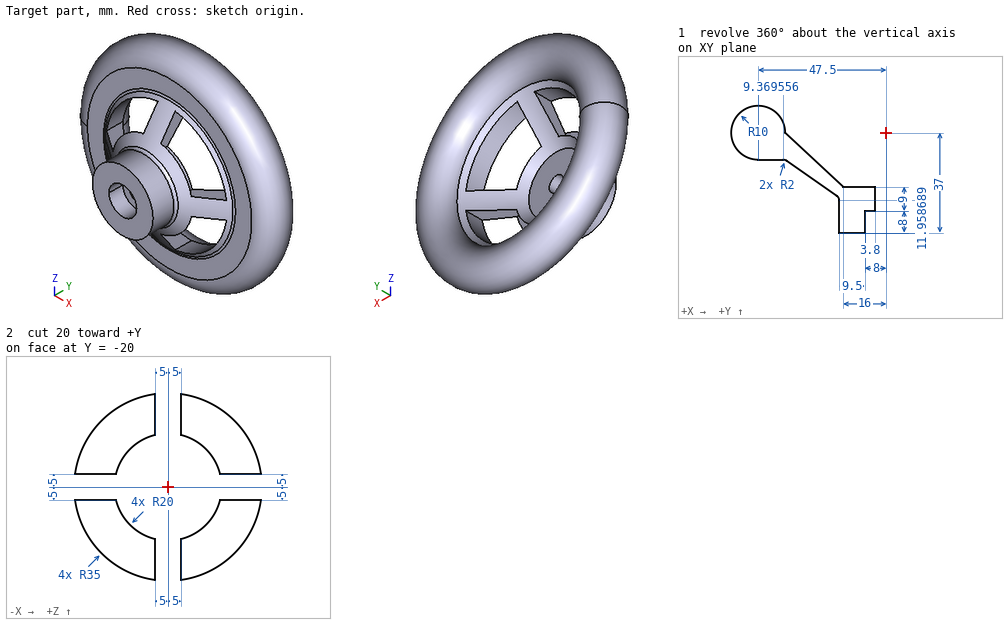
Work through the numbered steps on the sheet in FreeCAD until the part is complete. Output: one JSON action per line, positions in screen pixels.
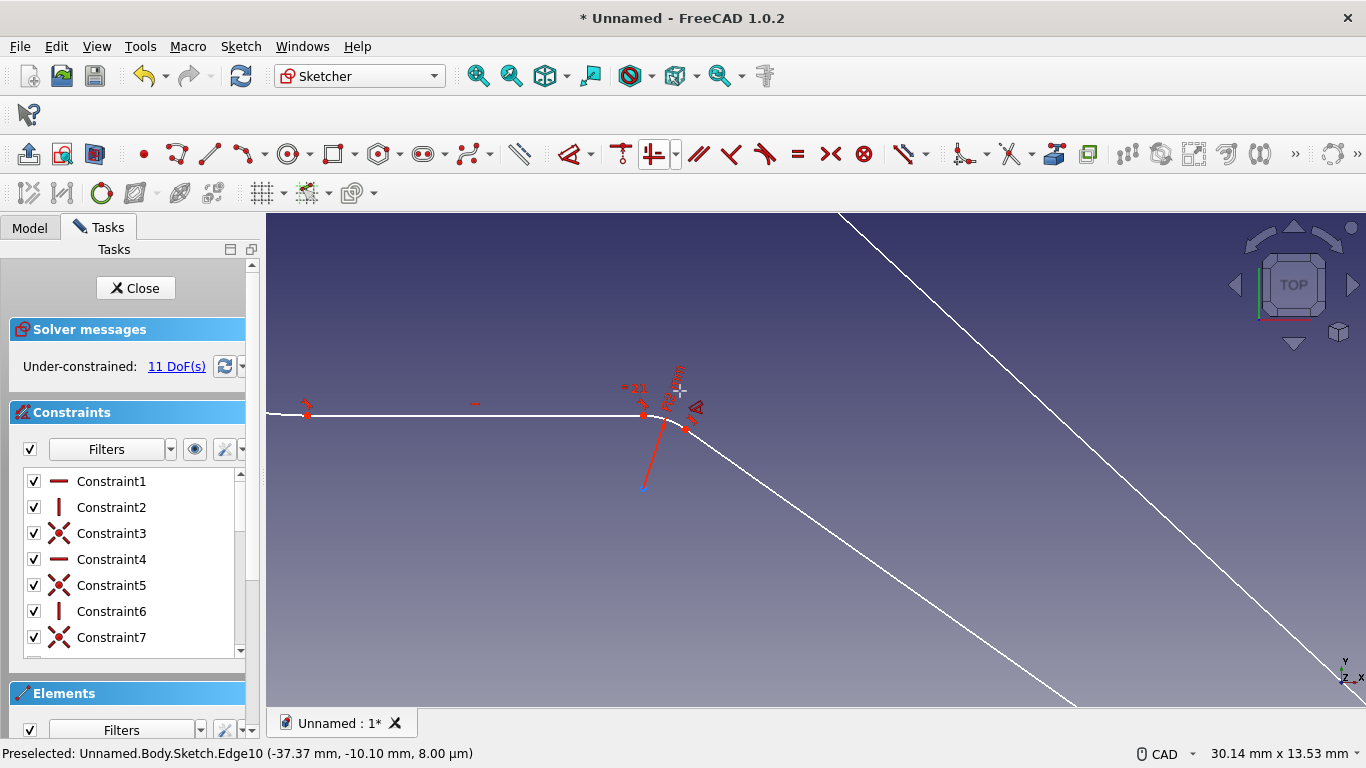
{"action": "scroll", "coordinate": [673, 424], "scroll_direction": "down", "scroll_amount": 8}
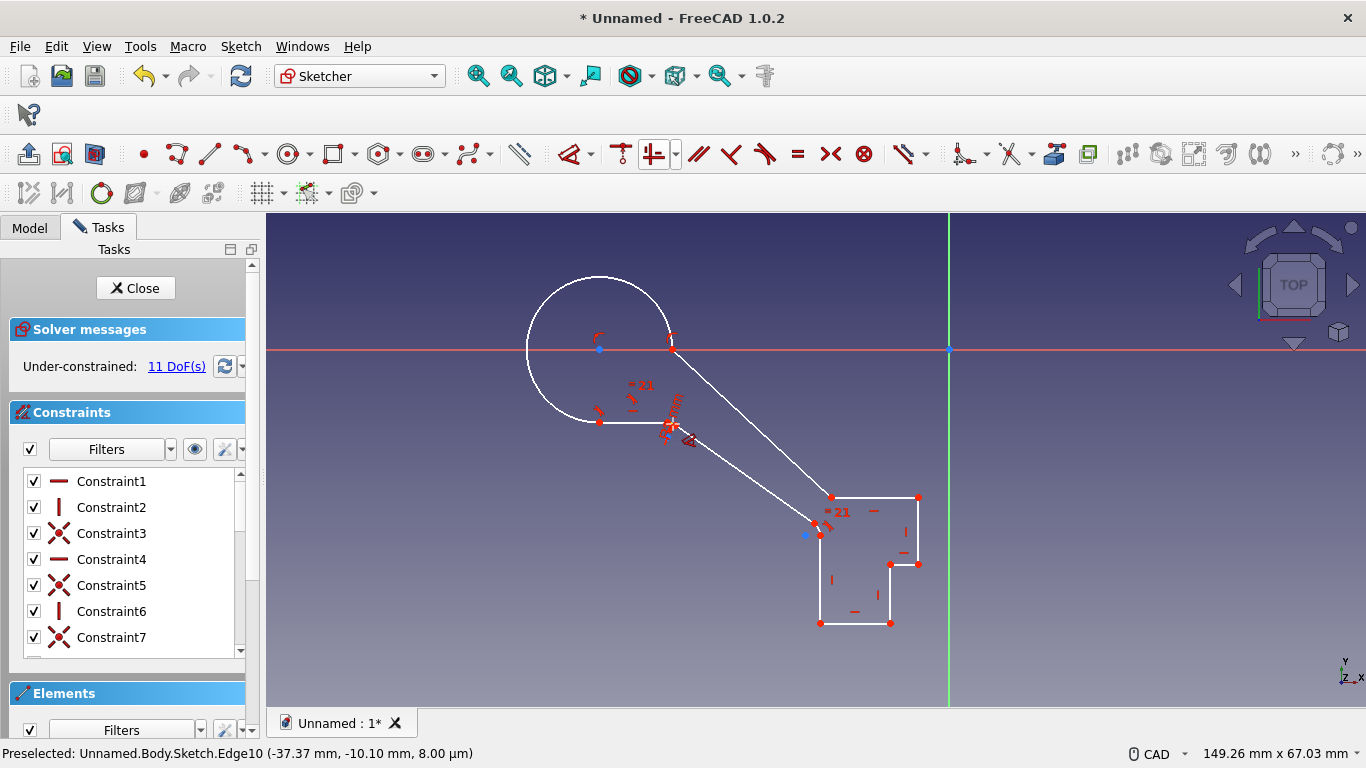
{"action": "left_click", "coordinate": [611, 278]}
{"action": "left_click", "coordinate": [616, 246]}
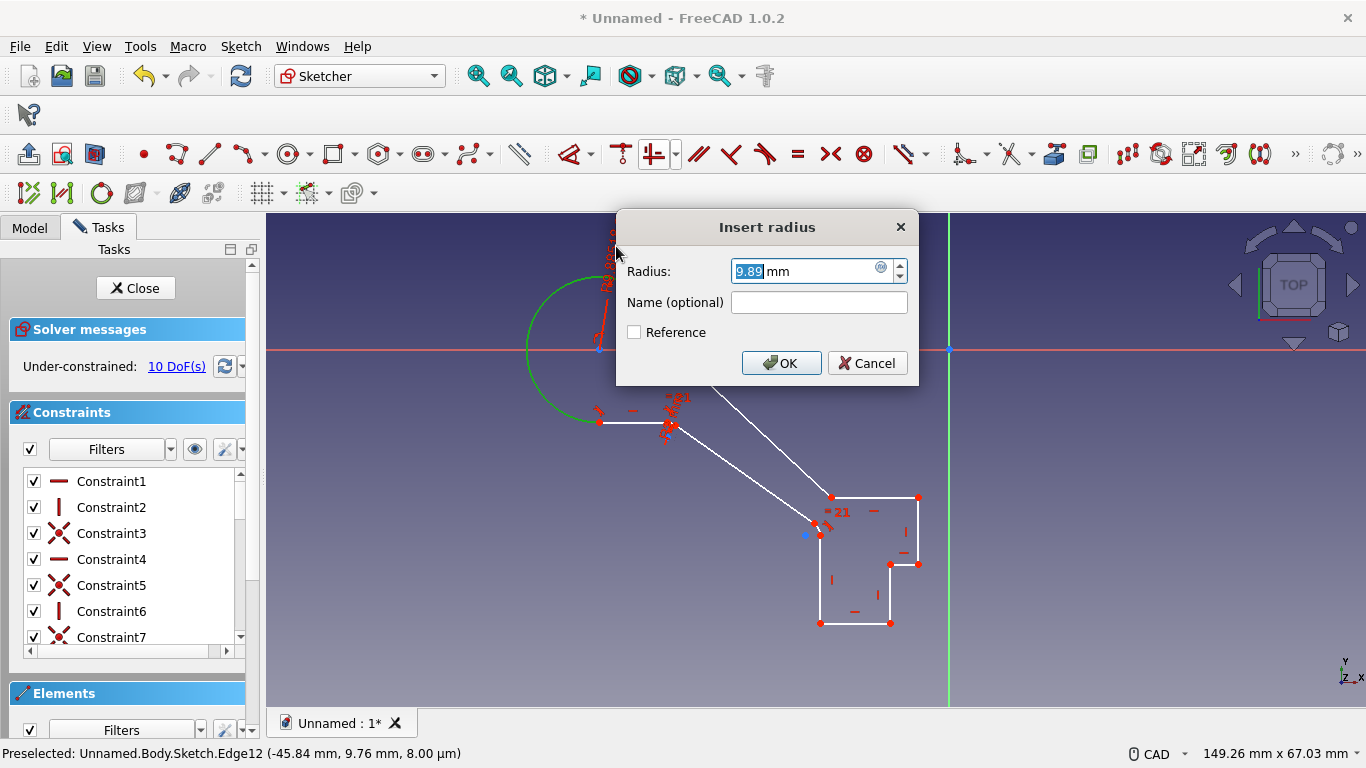
{"action": "type", "text": "10"}
{"action": "key", "text": "Return"}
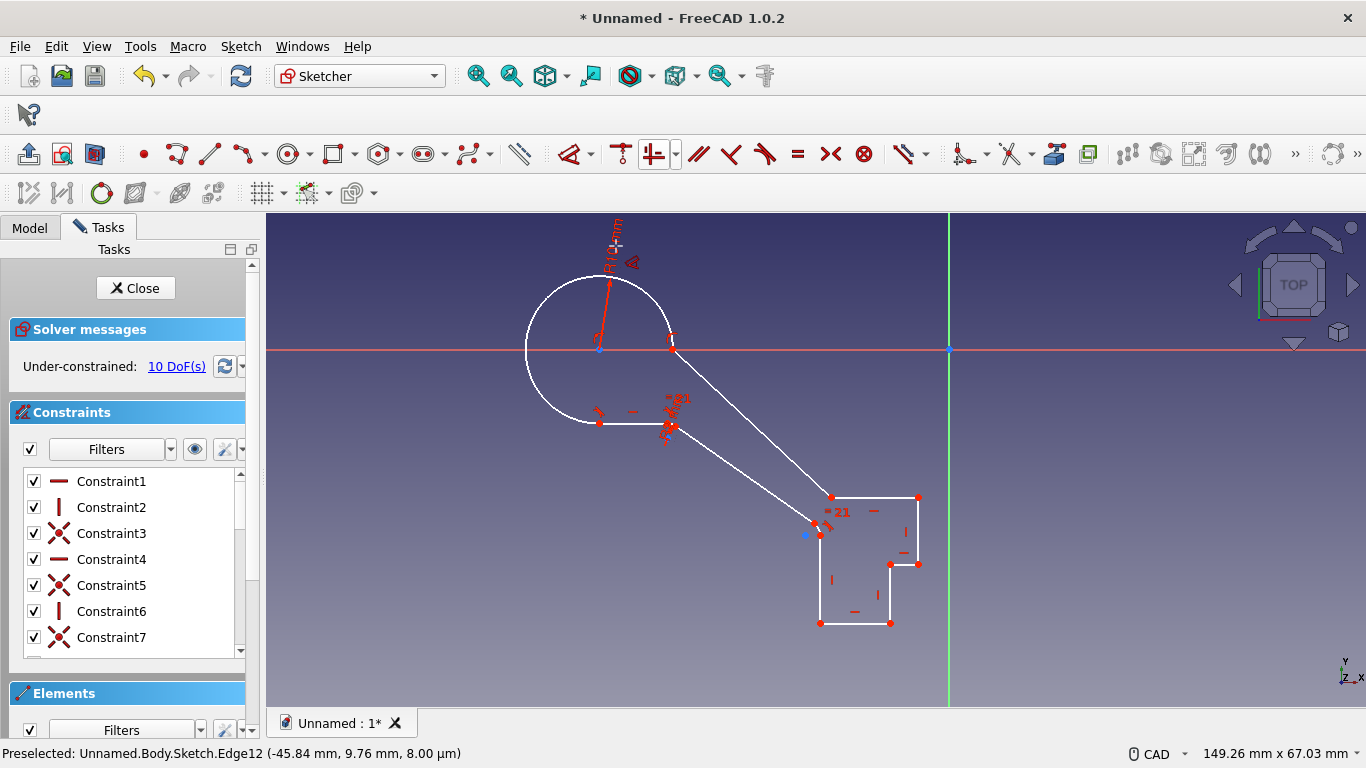
{"action": "left_click", "coordinate": [890, 606]}
{"action": "left_click", "coordinate": [924, 594]}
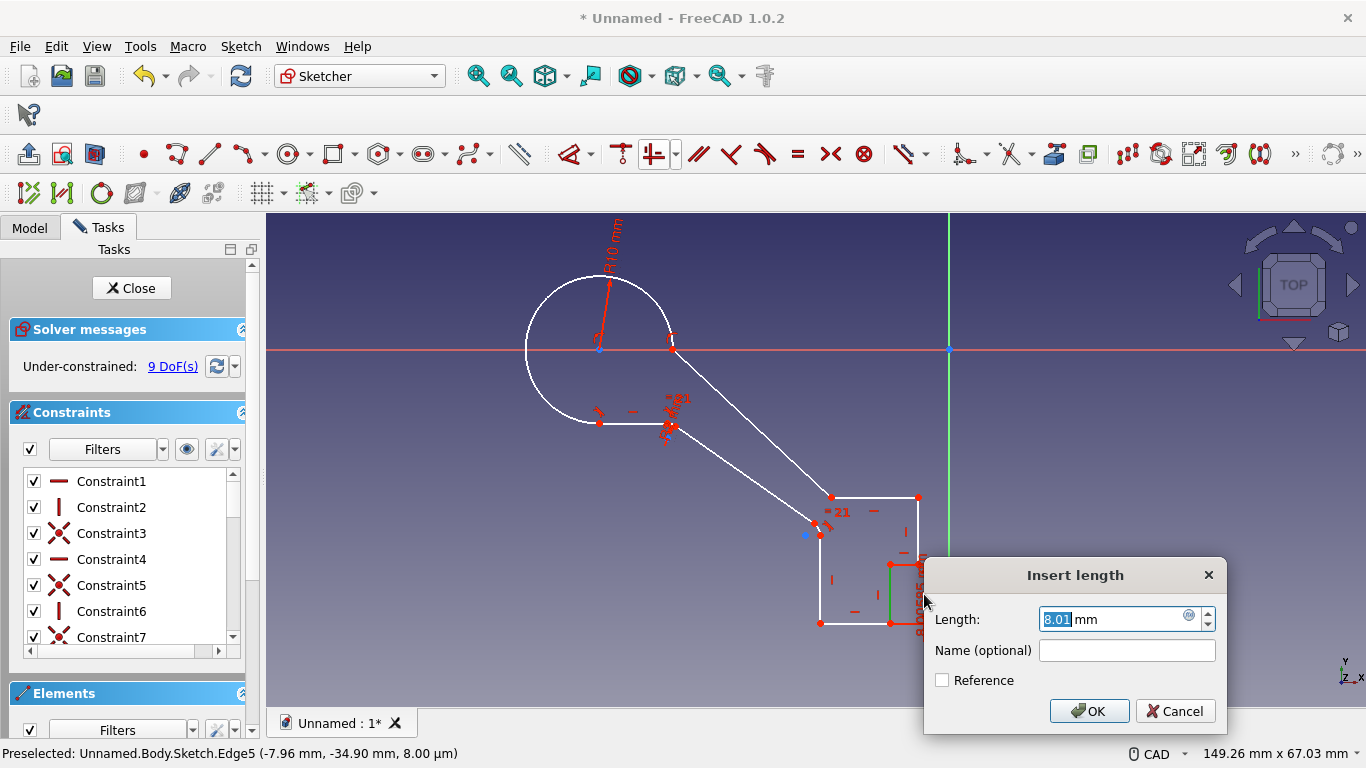
{"action": "type", "text": "8"}
{"action": "key", "text": "Return"}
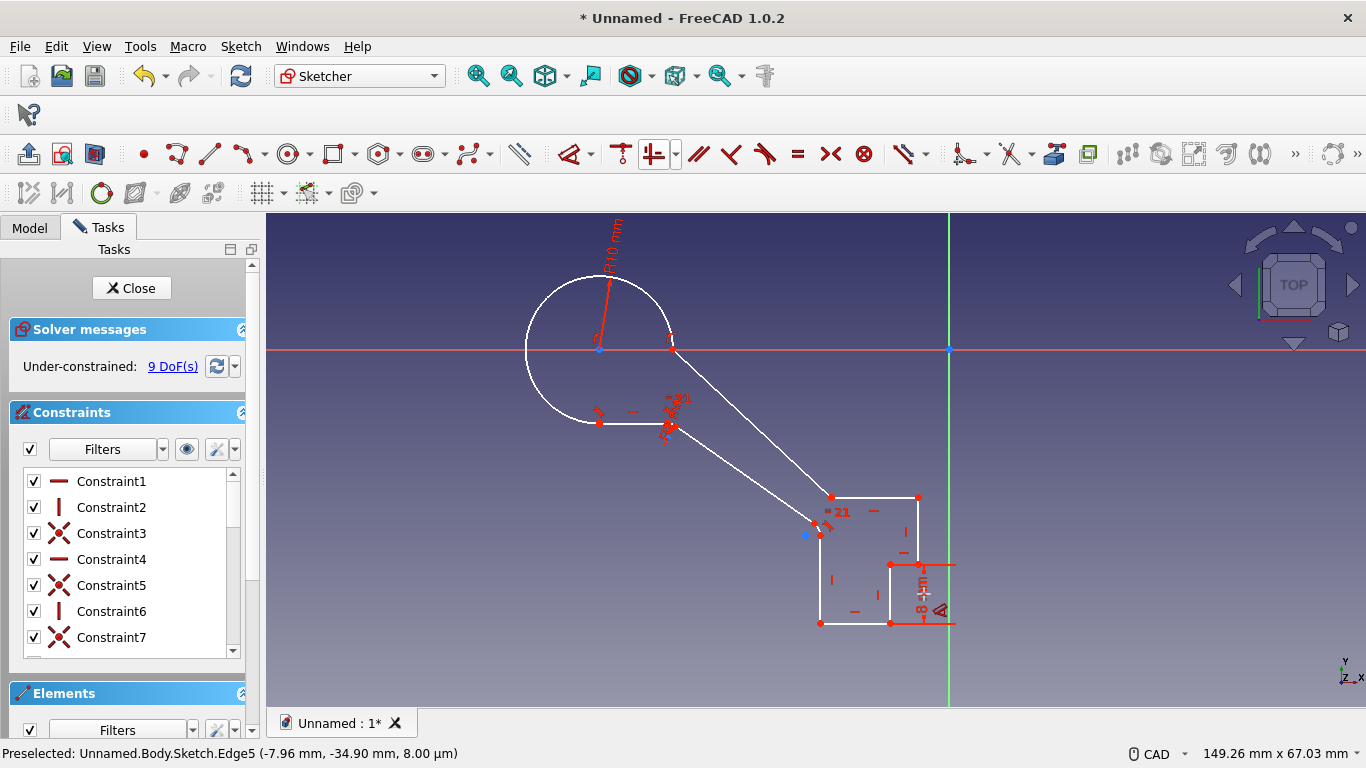
{"action": "left_click", "coordinate": [918, 545]}
{"action": "left_click", "coordinate": [884, 531]}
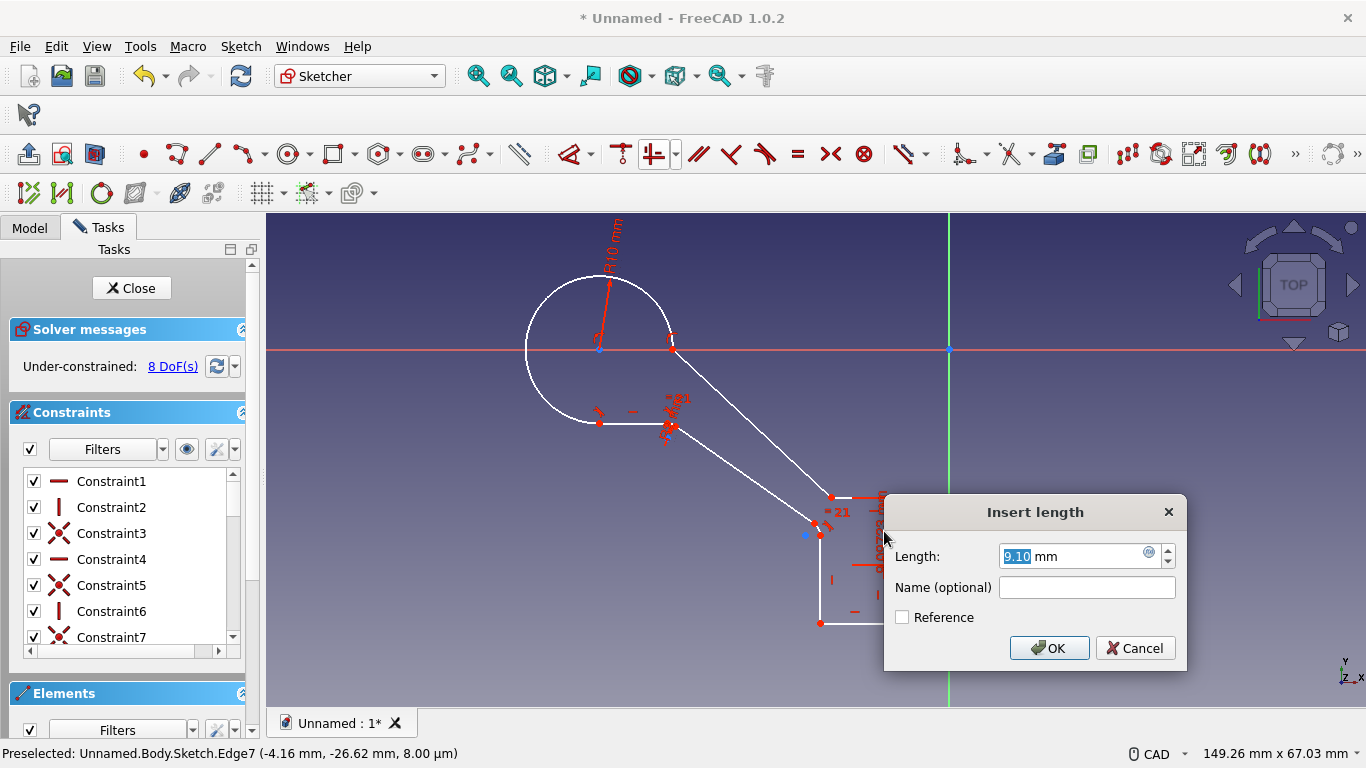
{"action": "type", "text": "9"}
{"action": "key", "text": "Return"}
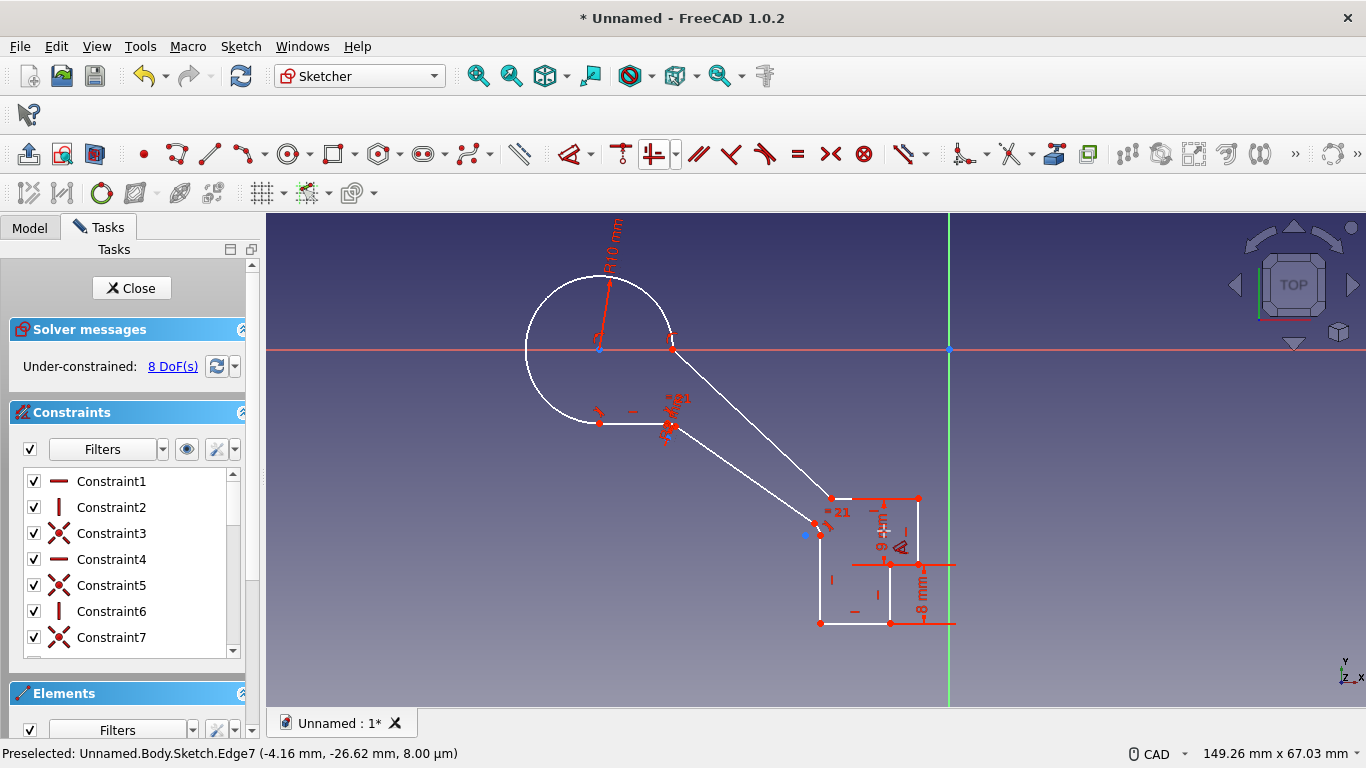
{"action": "left_click", "coordinate": [890, 624]}
{"action": "left_click", "coordinate": [920, 658]}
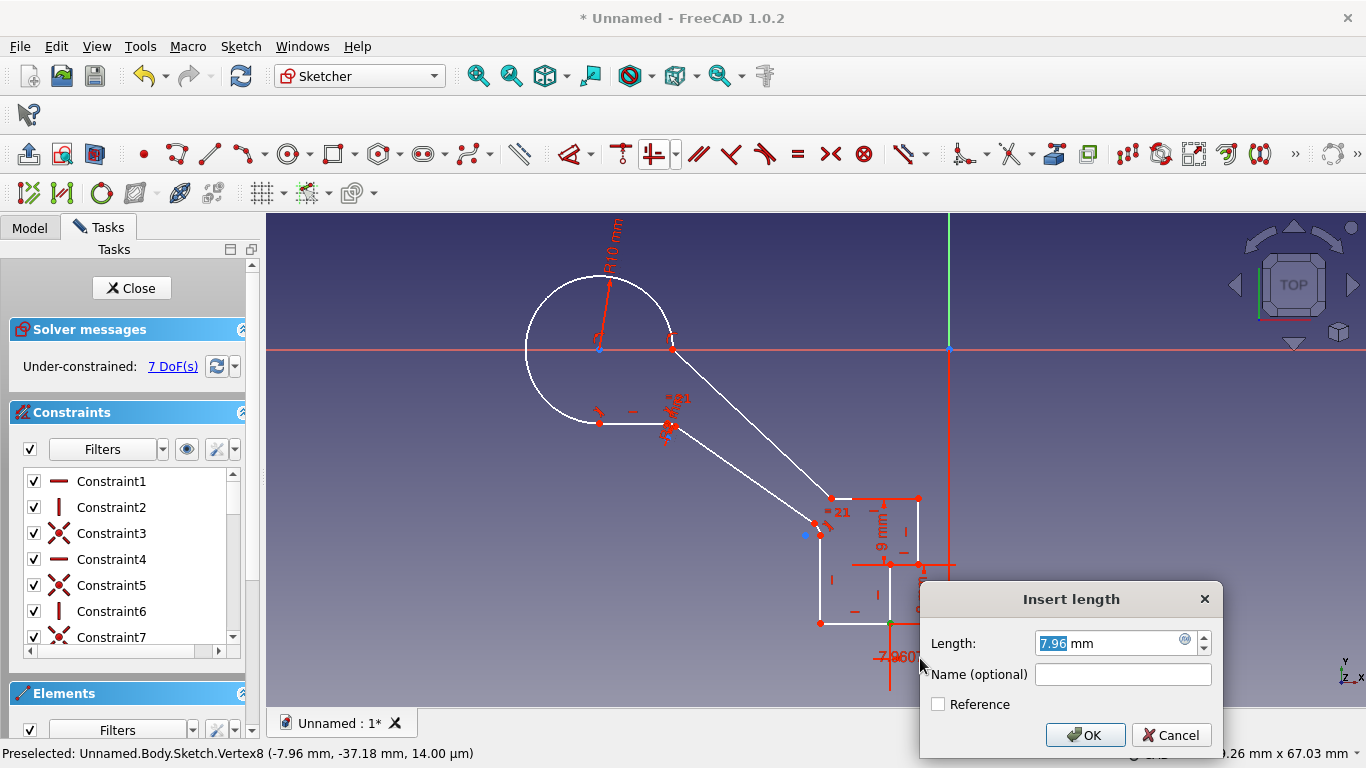
{"action": "type", "text": "8"}
{"action": "key", "text": "Return"}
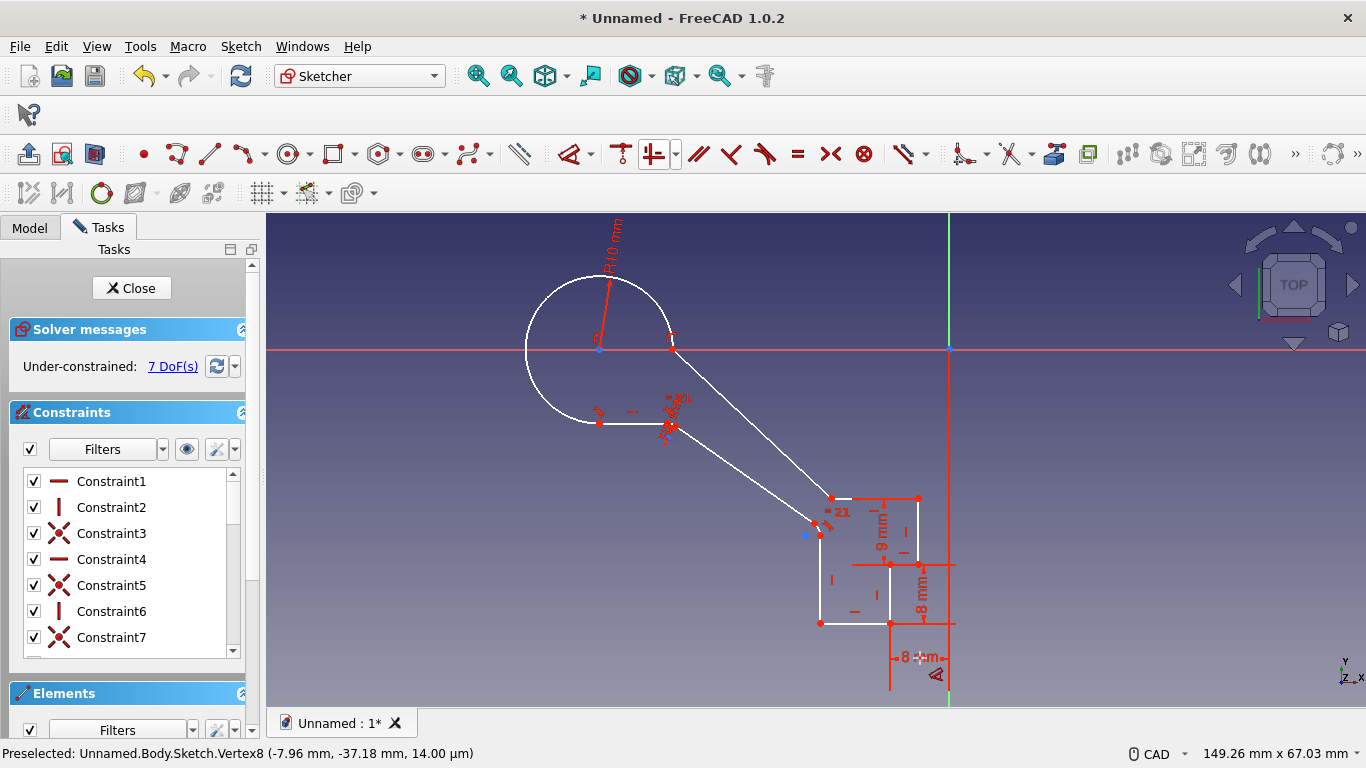
{"action": "left_click", "coordinate": [841, 624]}
{"action": "left_click", "coordinate": [839, 658]}